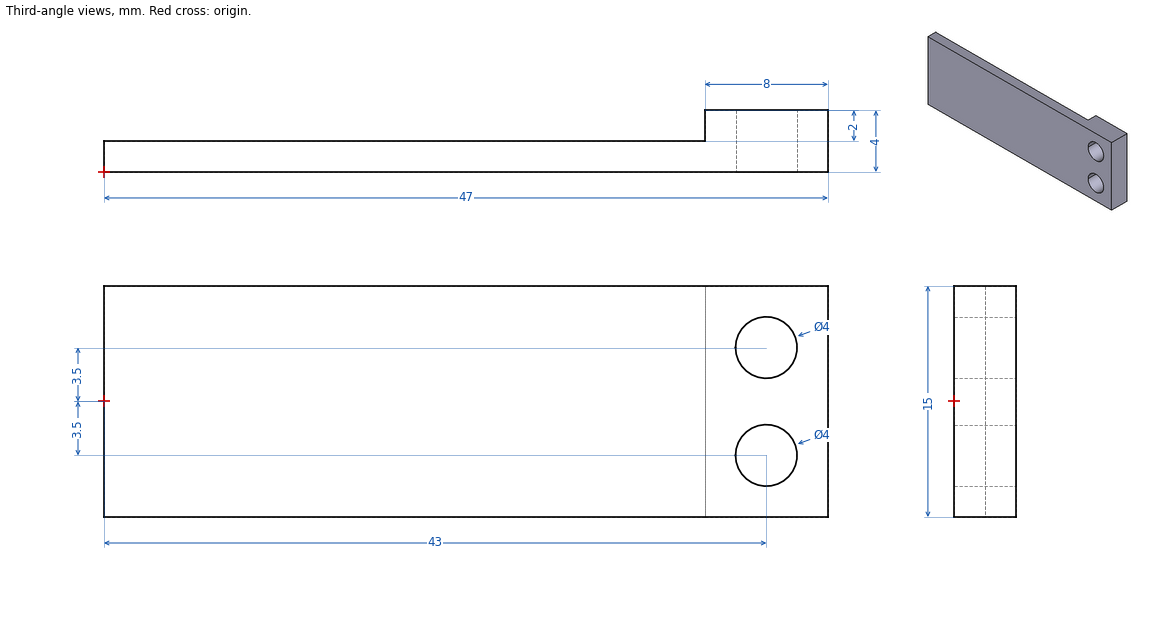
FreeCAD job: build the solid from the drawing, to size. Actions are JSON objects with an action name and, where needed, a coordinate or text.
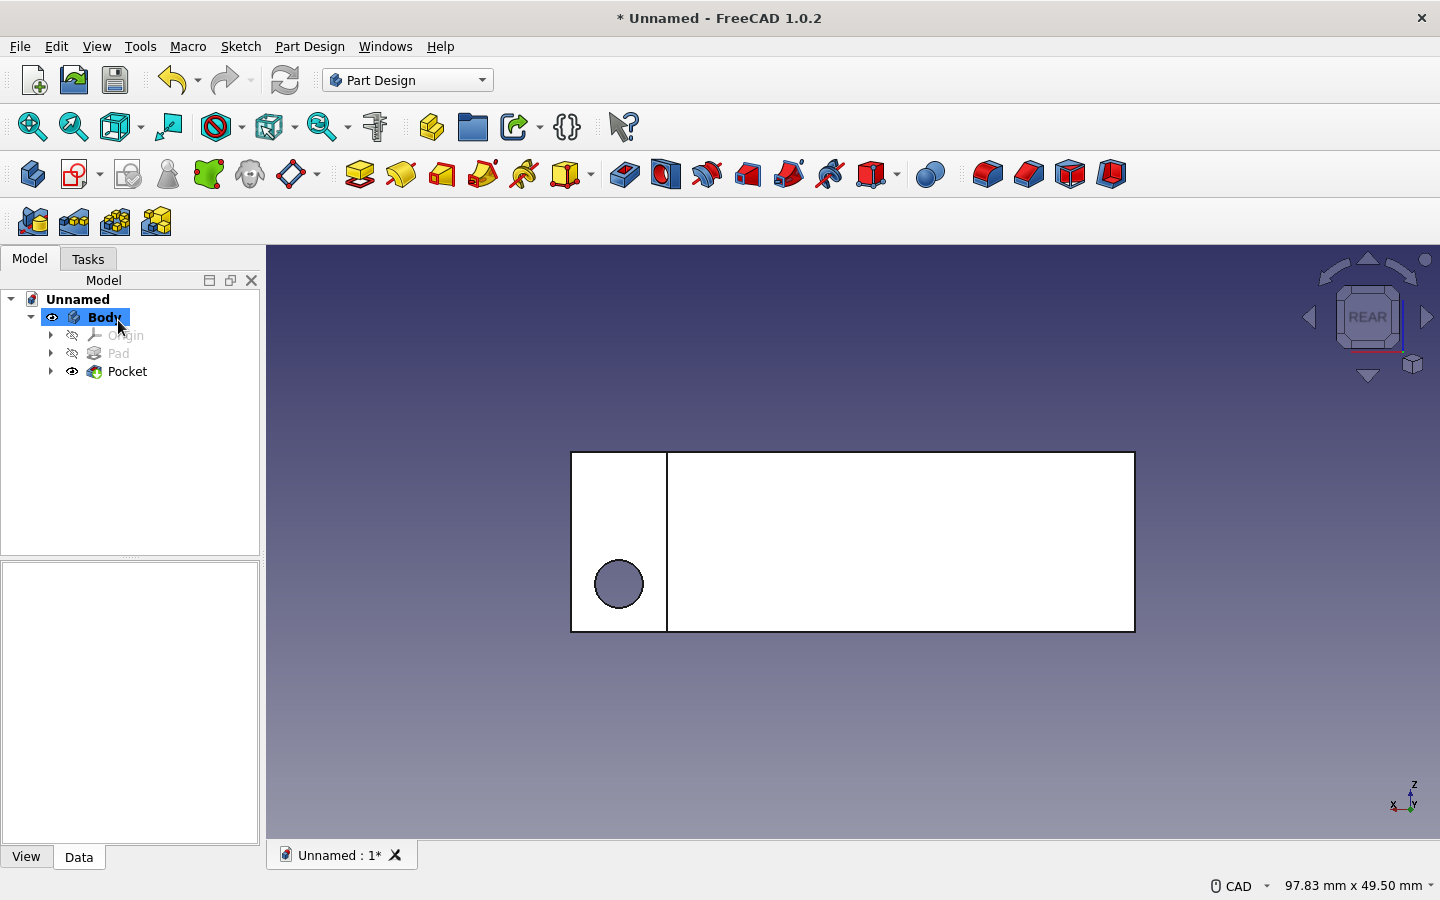
{"action": "left_click", "coordinate": [619, 515]}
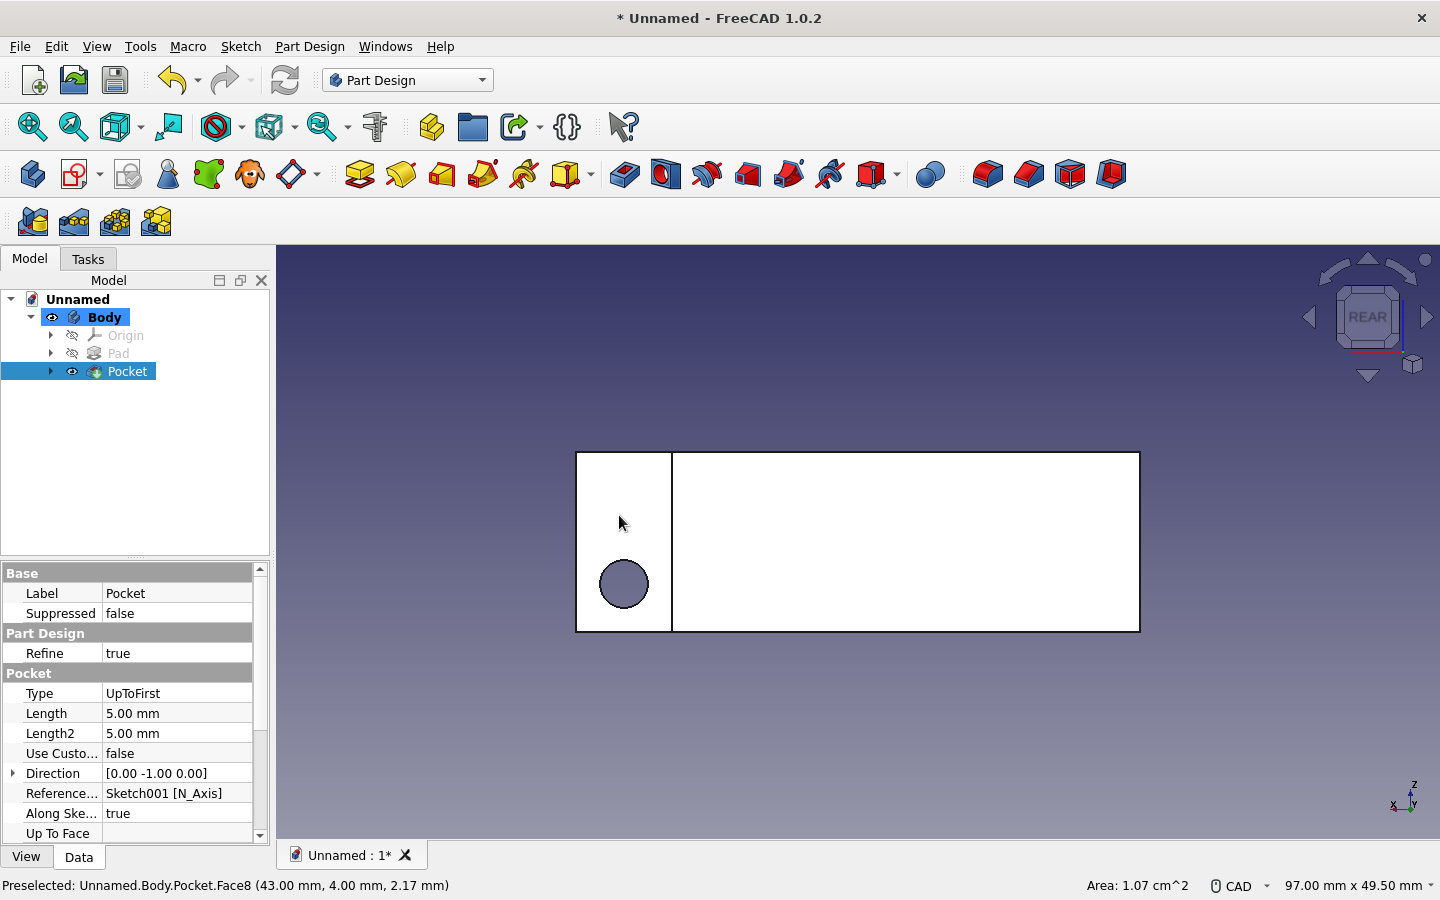
{"action": "left_click", "coordinate": [74, 174]}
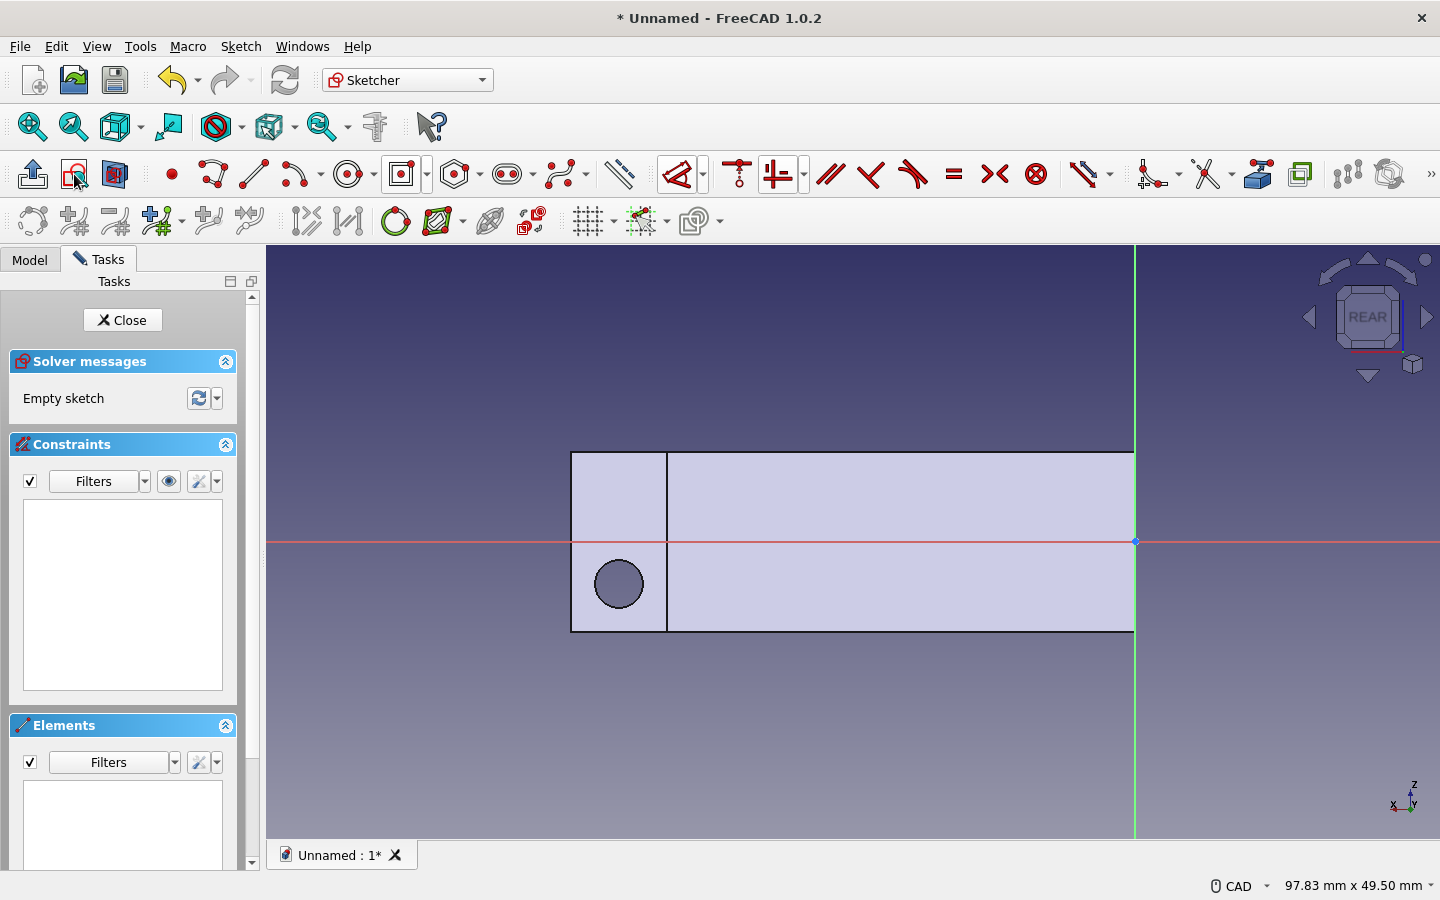
{"action": "scroll", "coordinate": [593, 493], "scroll_direction": "up", "scroll_amount": 10}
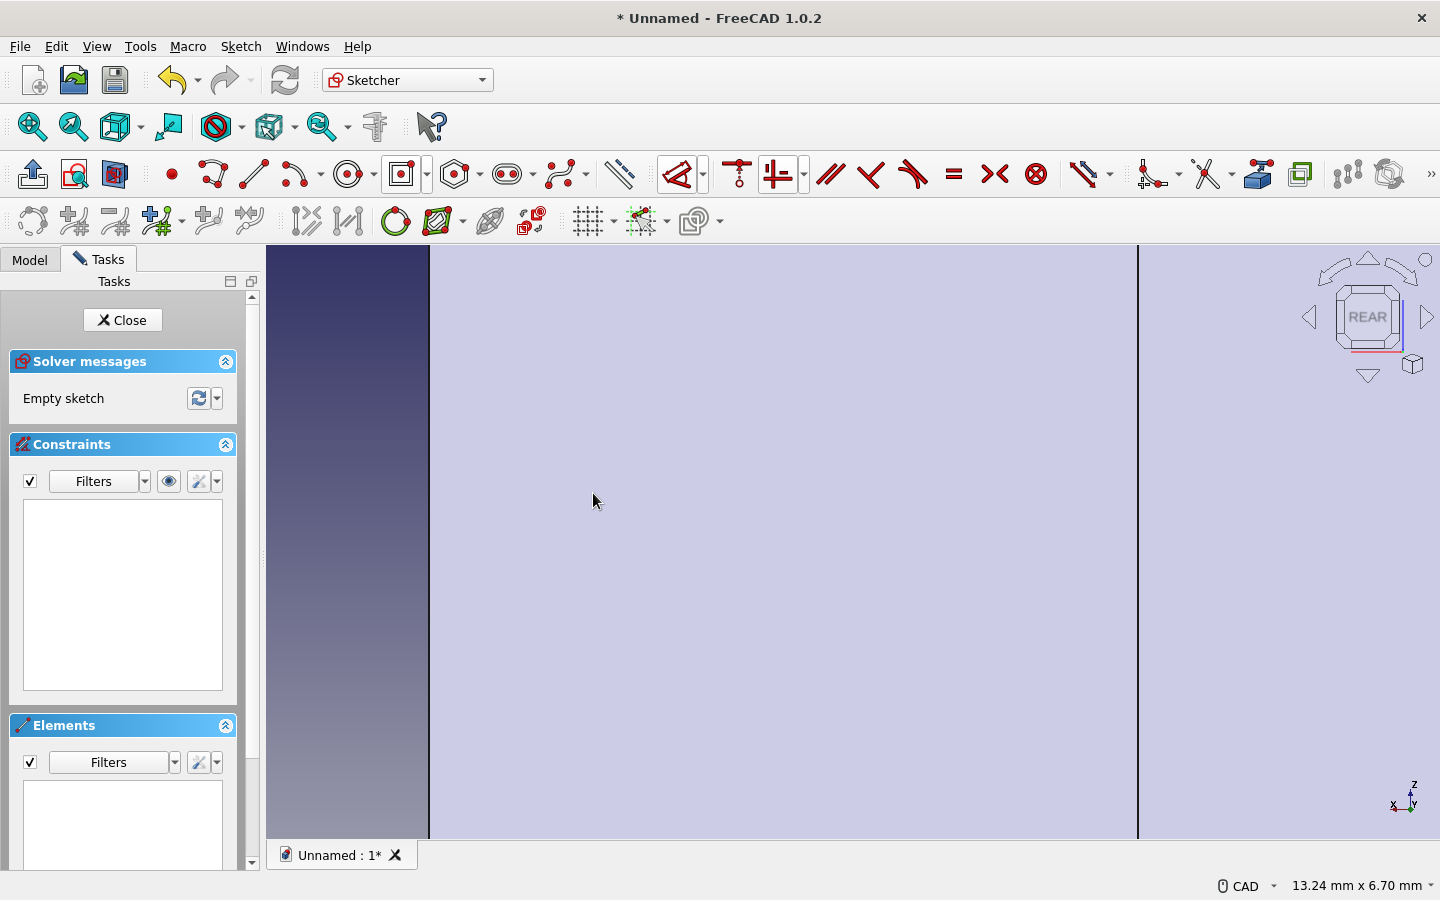
{"action": "left_click", "coordinate": [348, 174]}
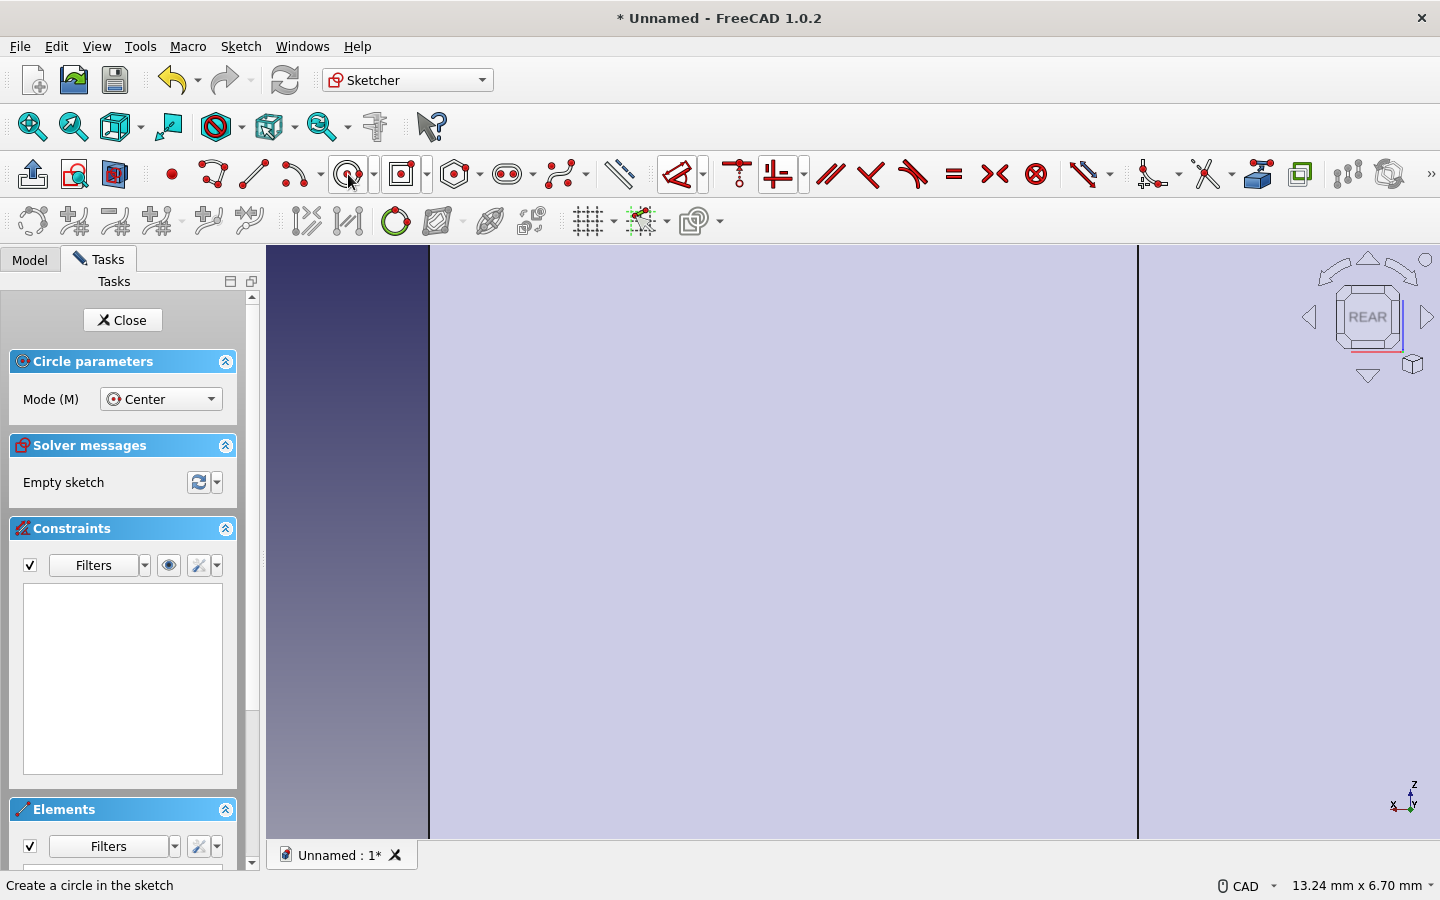
{"action": "left_click", "coordinate": [783, 542]}
{"action": "left_click", "coordinate": [909, 417]}
{"action": "key", "text": "Escape"}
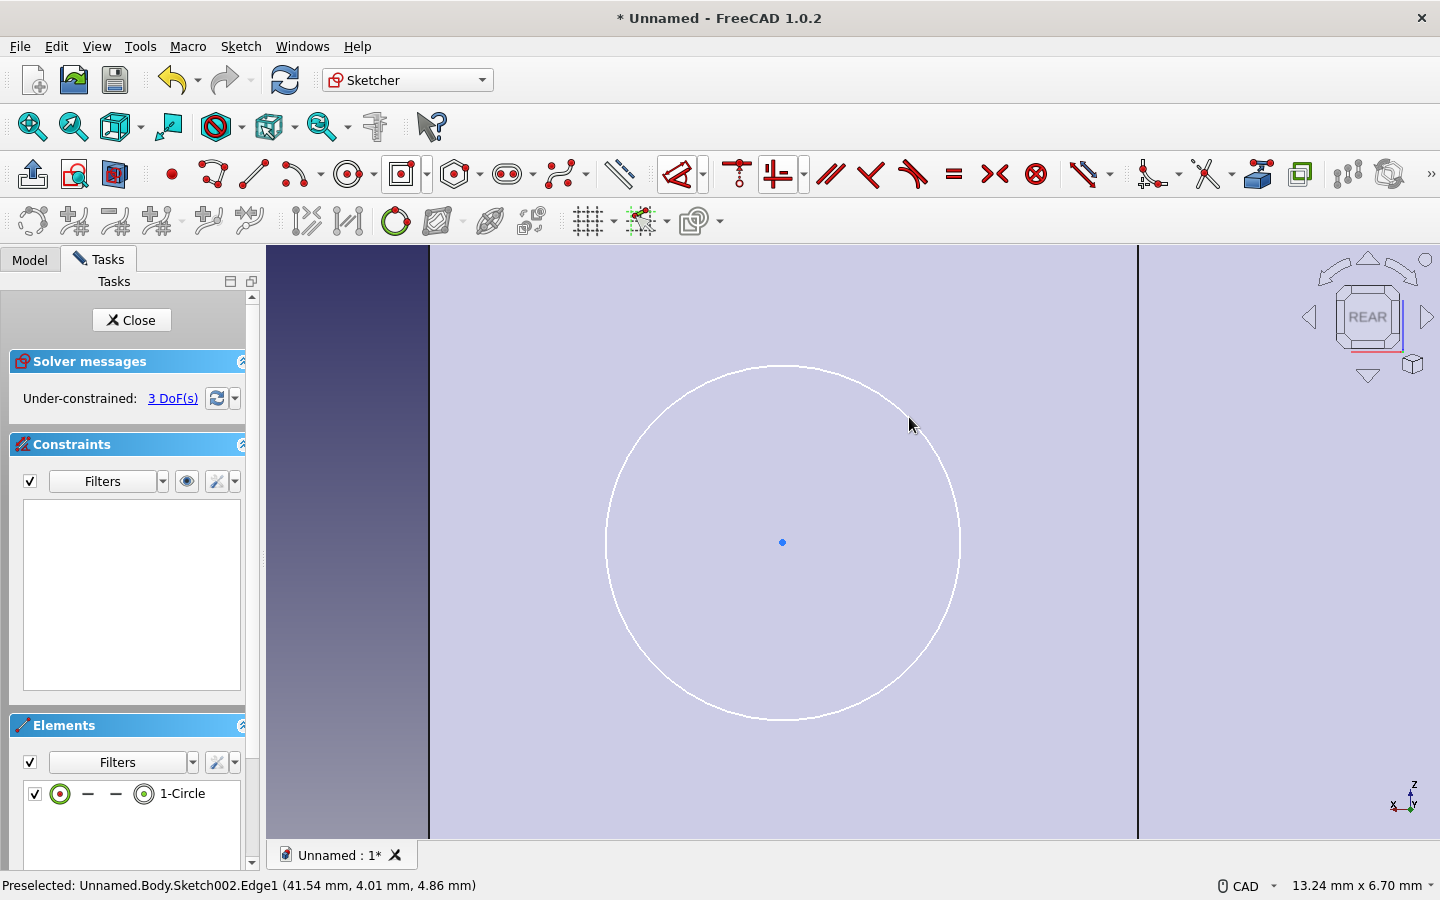
{"action": "left_click", "coordinate": [908, 417]}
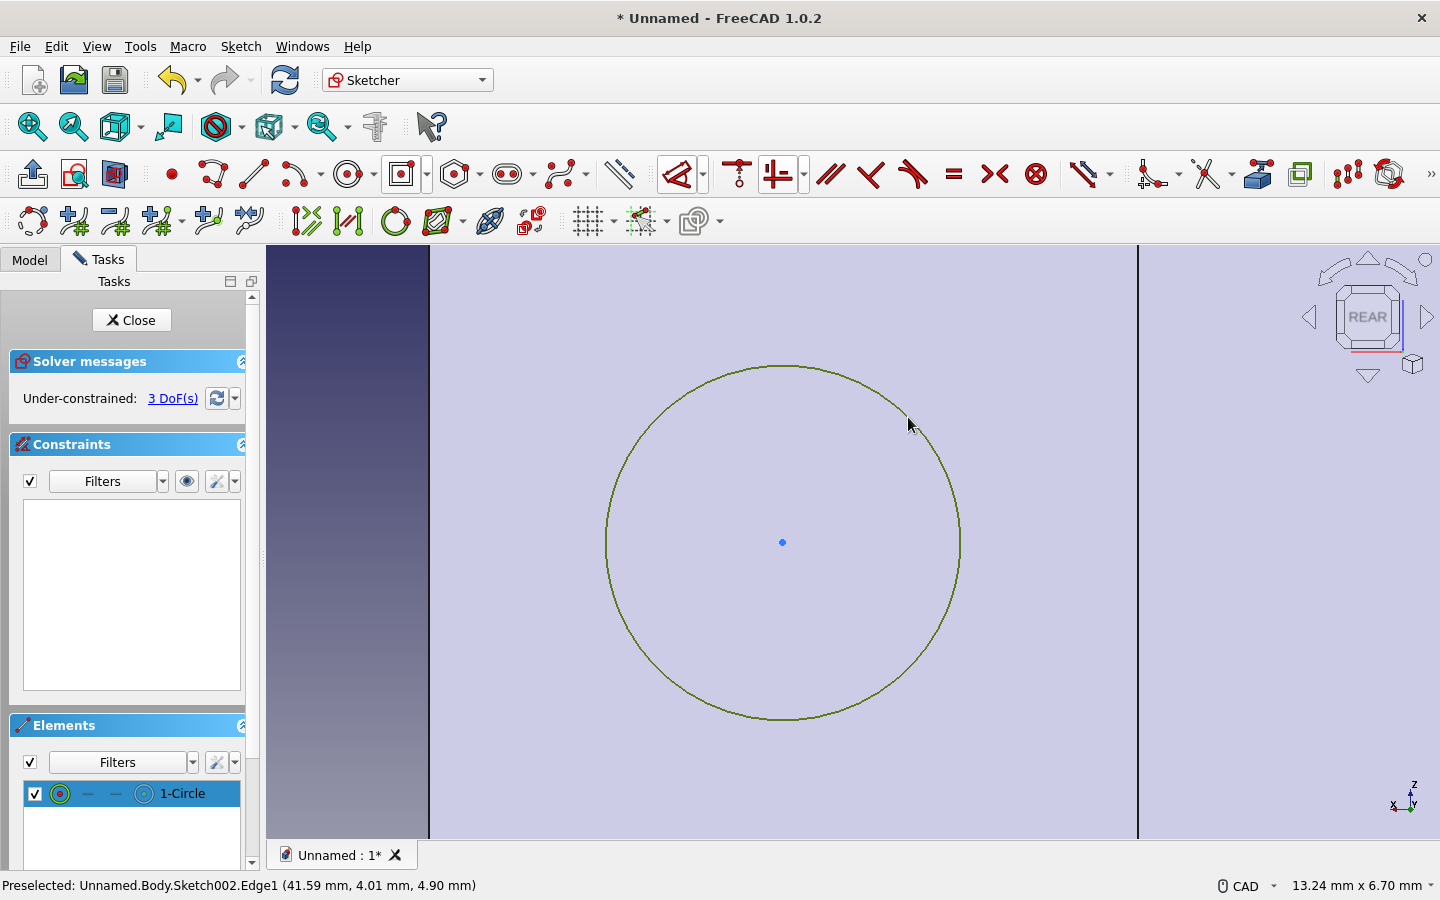
{"action": "key", "text": "k o"}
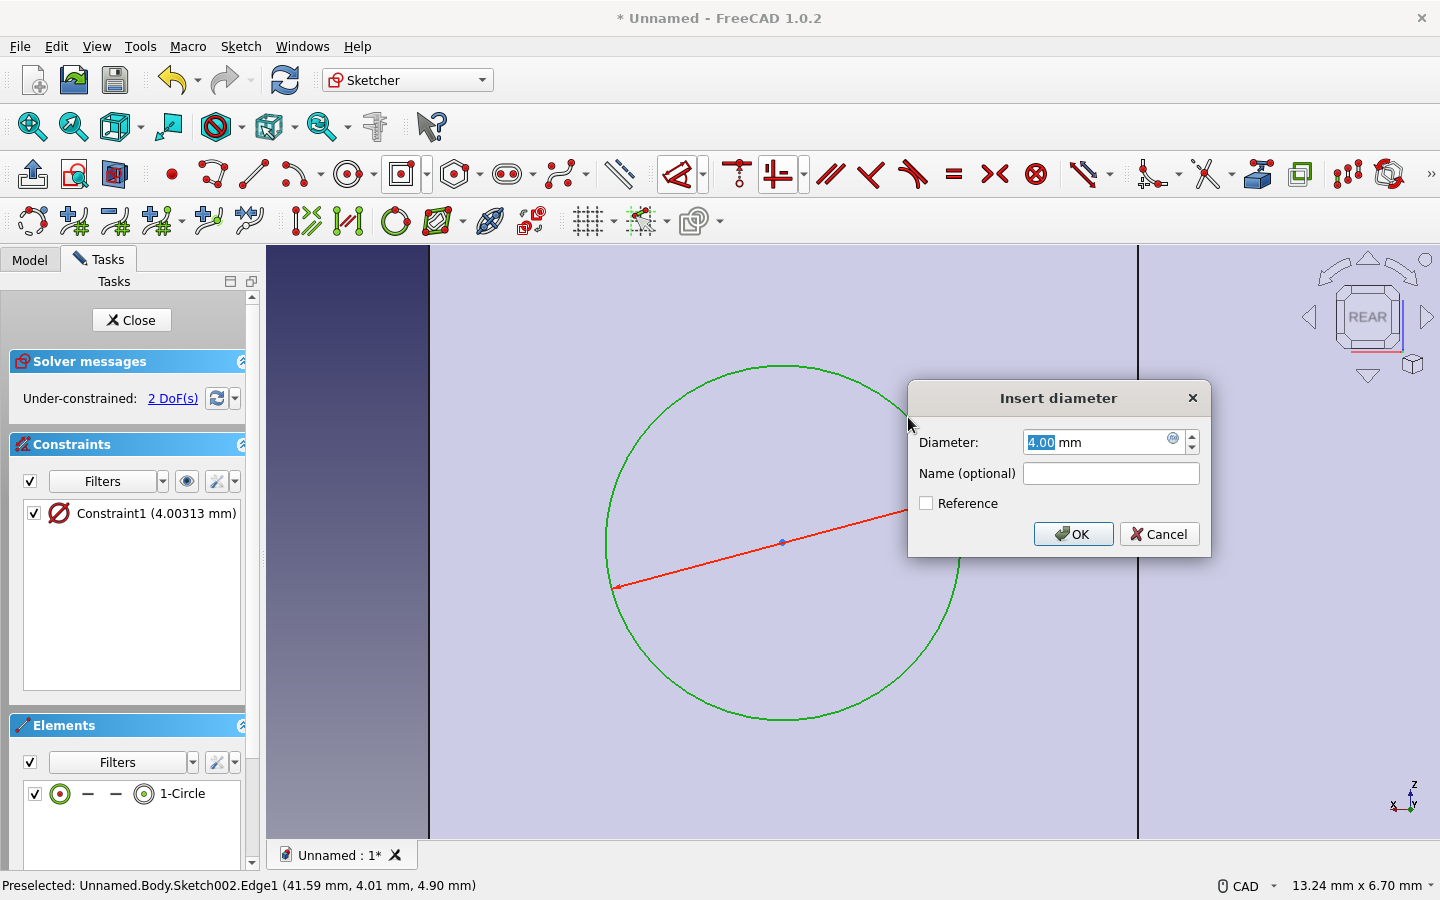
{"action": "type", "text": "4"}
{"action": "key", "text": "Return"}